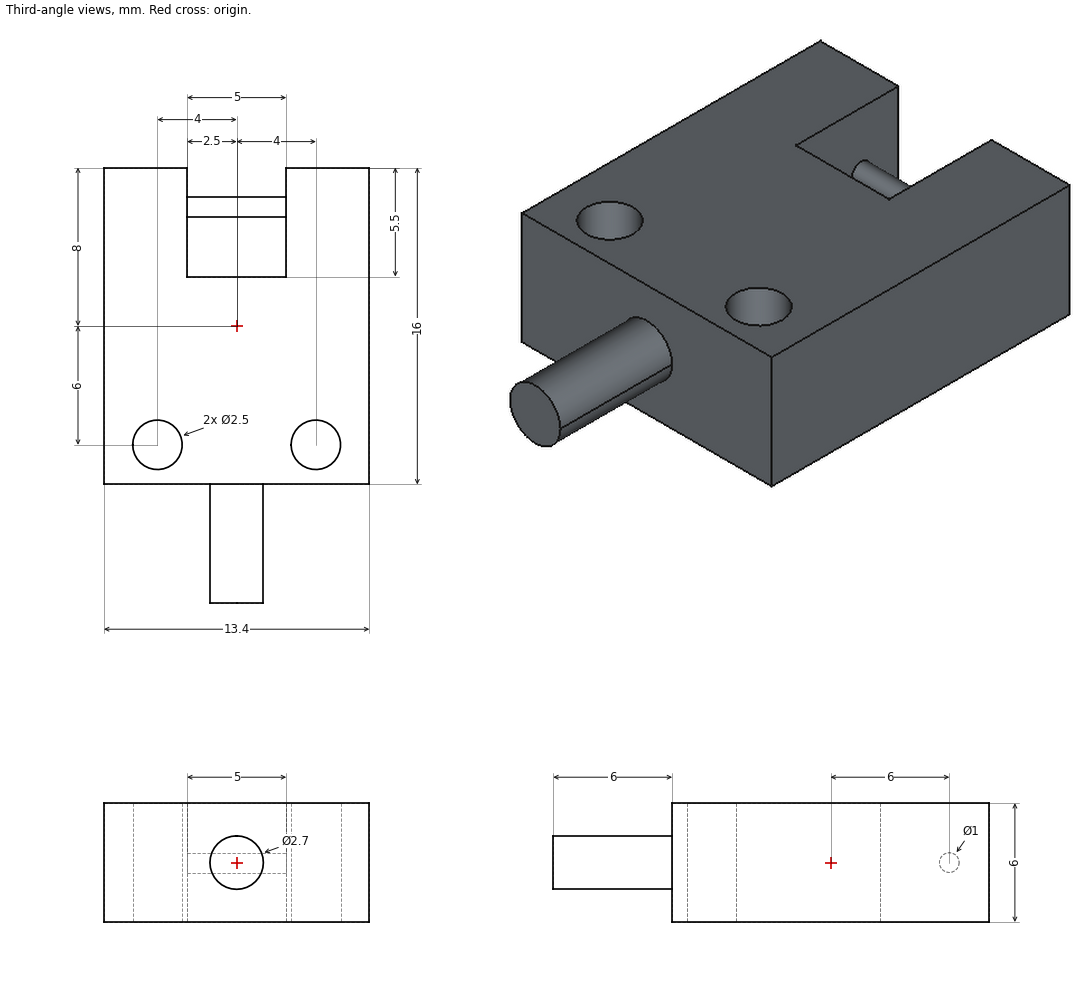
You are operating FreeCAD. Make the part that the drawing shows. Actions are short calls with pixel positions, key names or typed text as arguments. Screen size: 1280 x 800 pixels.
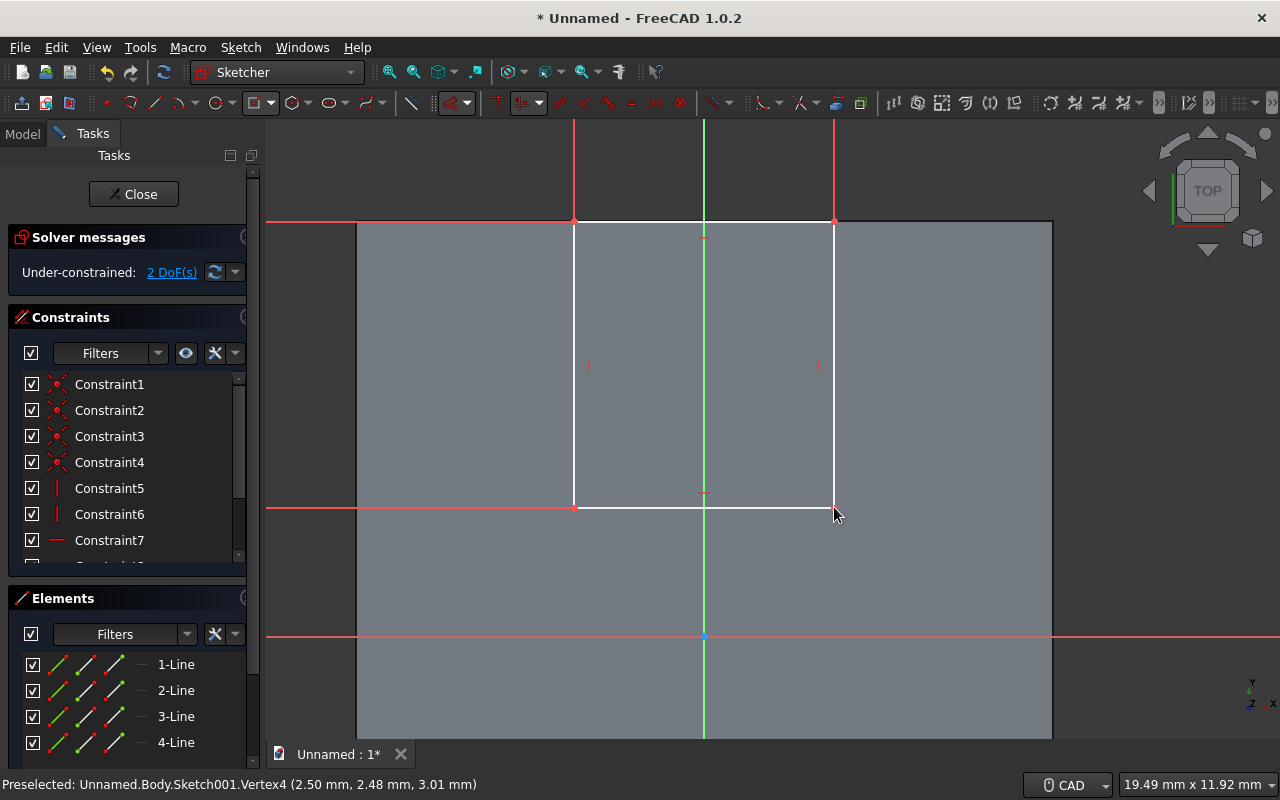
click(450, 104)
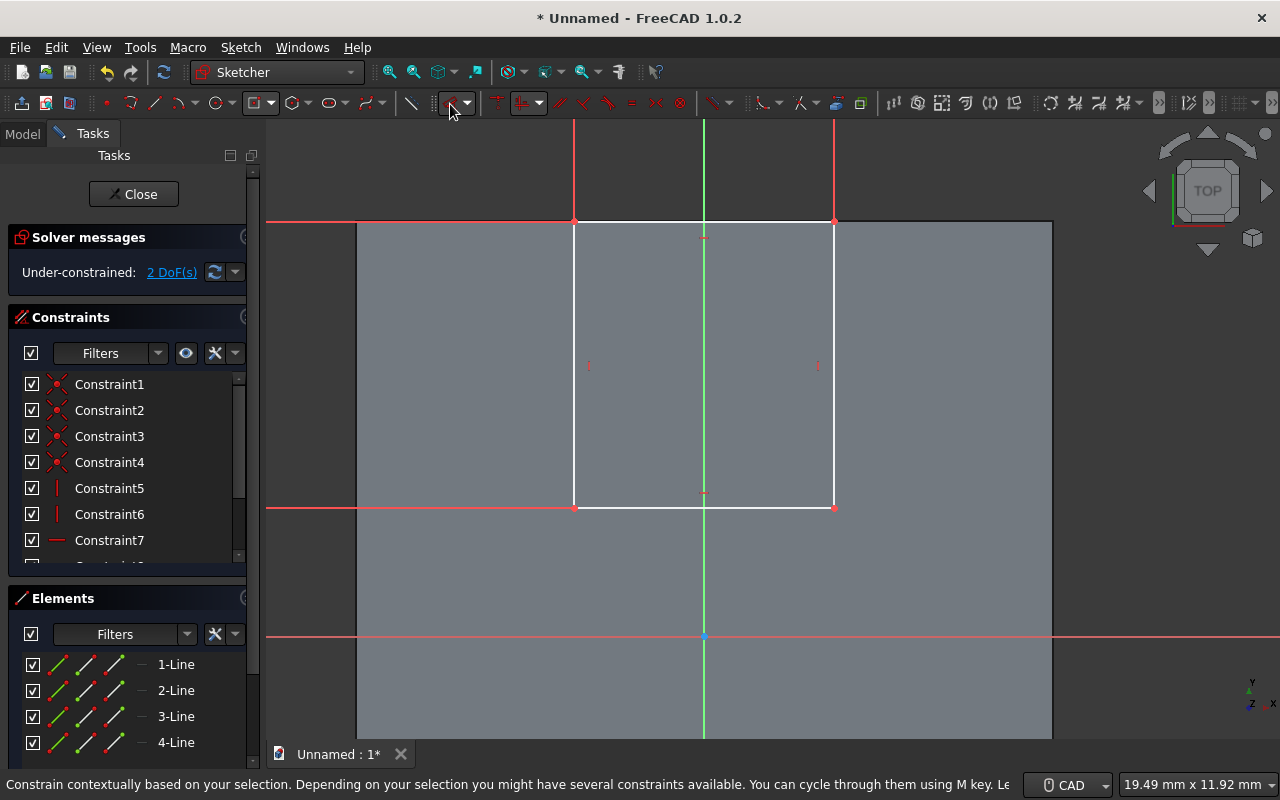
click(574, 222)
click(540, 429)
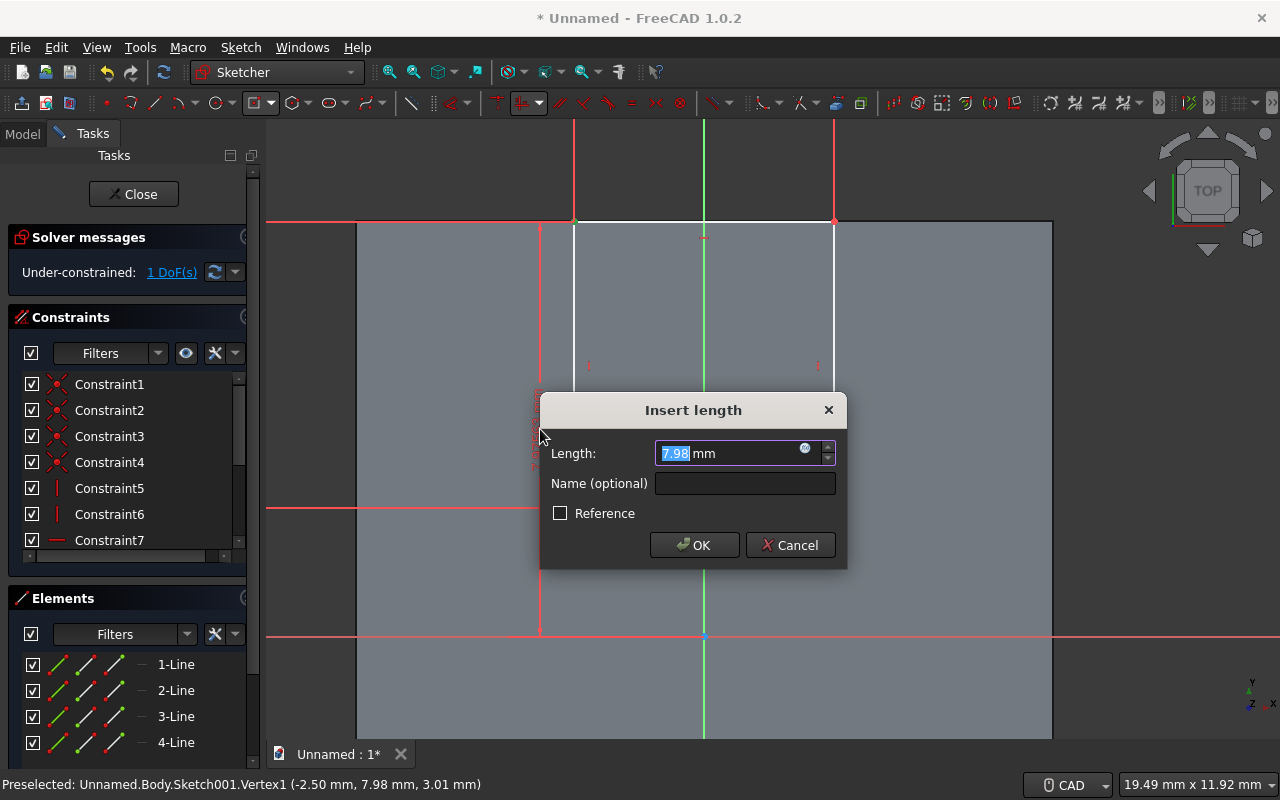
text(8)
key(Return)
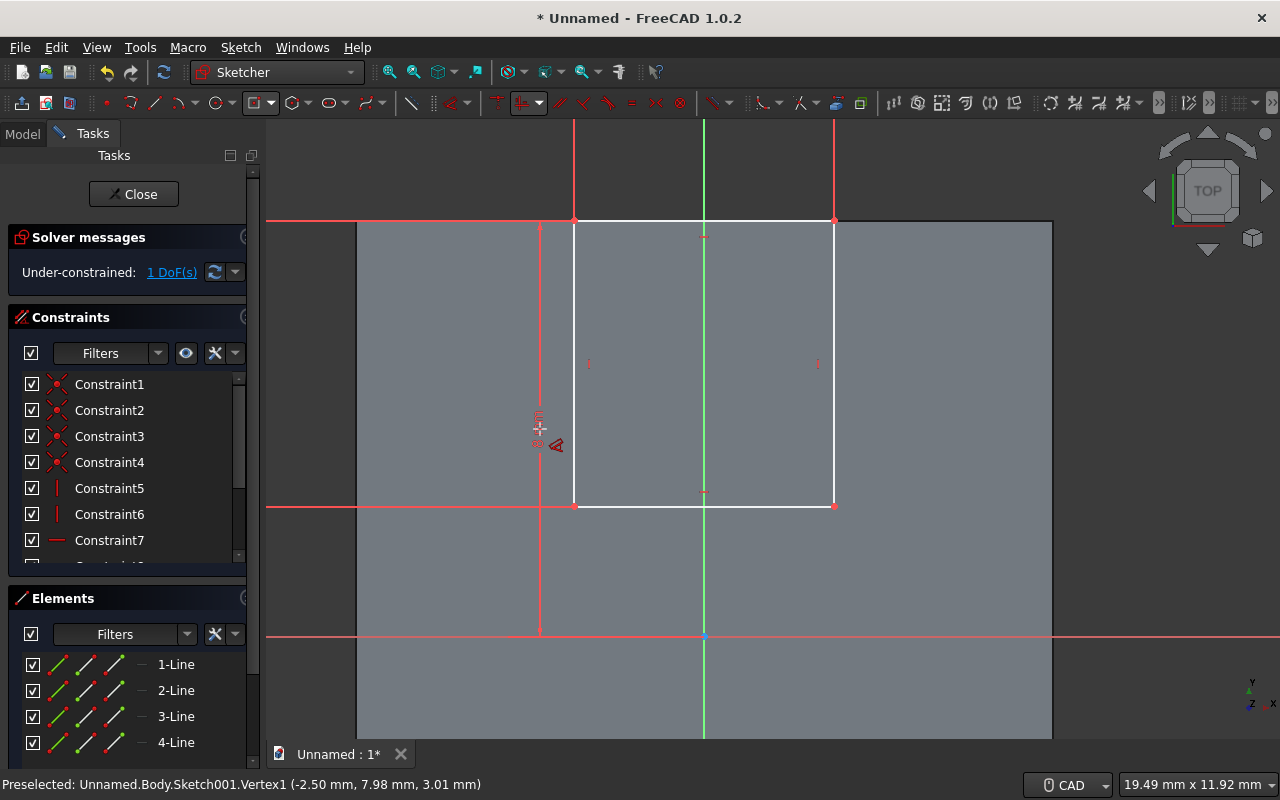
click(574, 221)
click(639, 671)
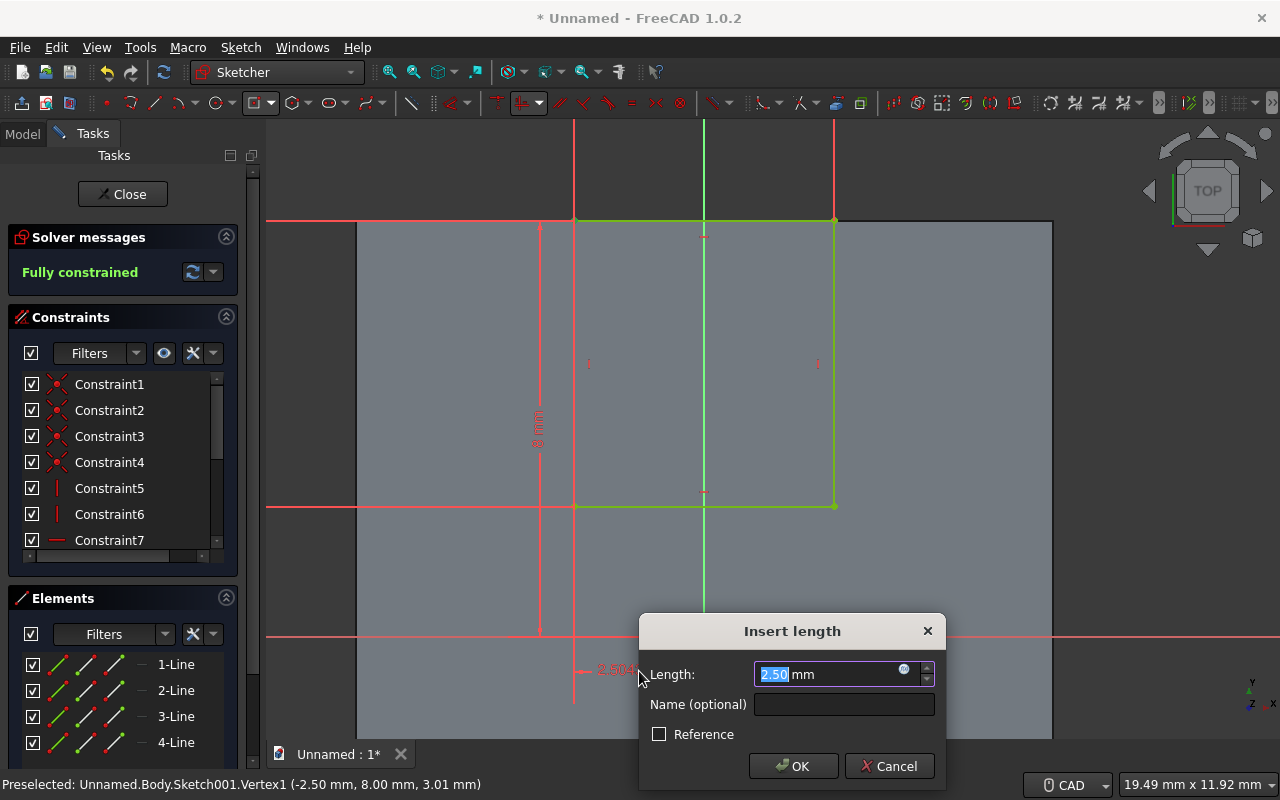
text(2.5)
key(Return)
key(Escape)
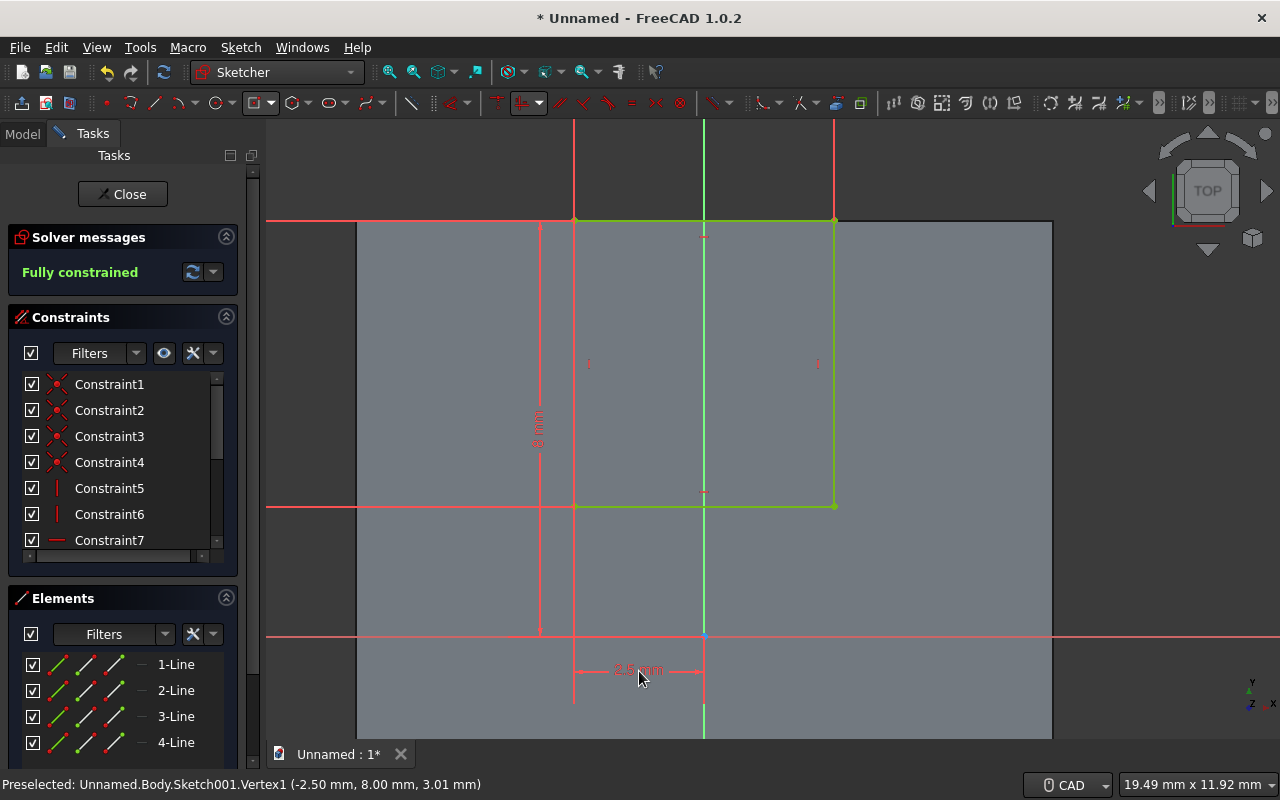
click(123, 194)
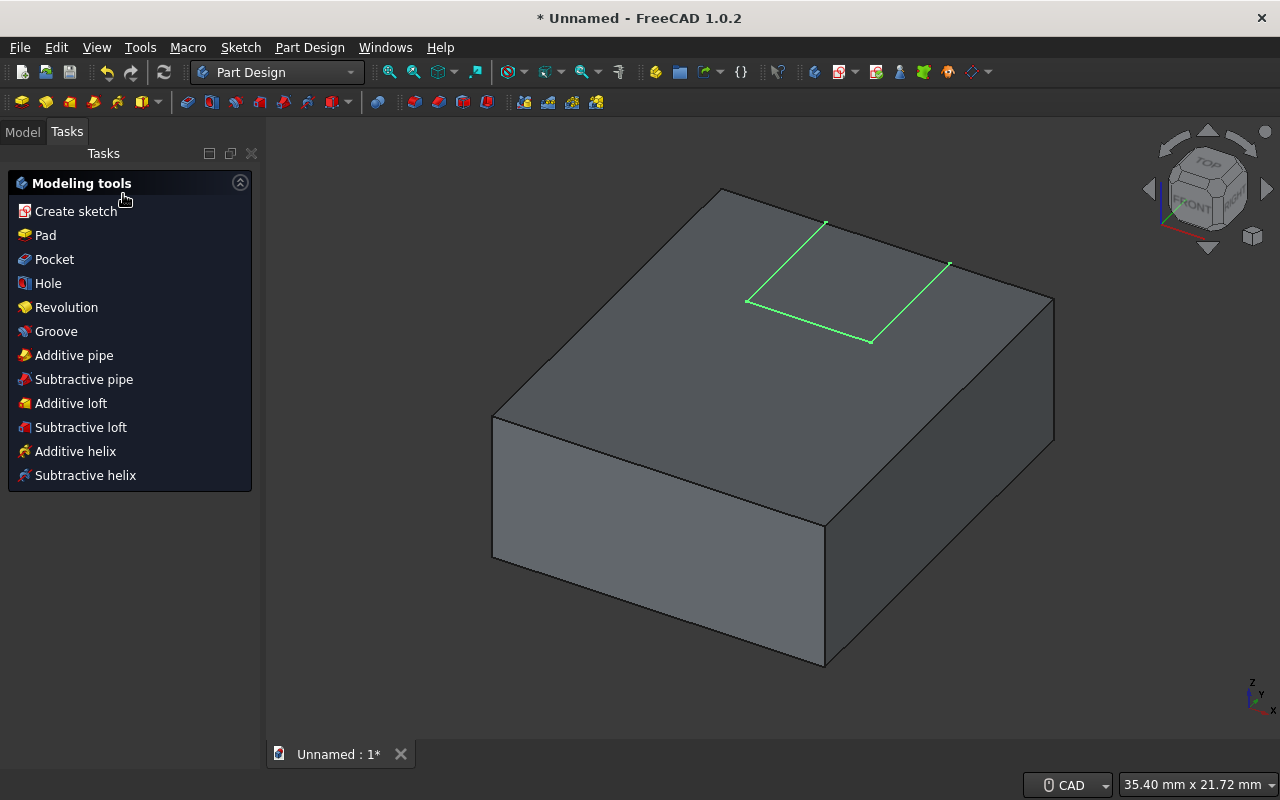
click(188, 102)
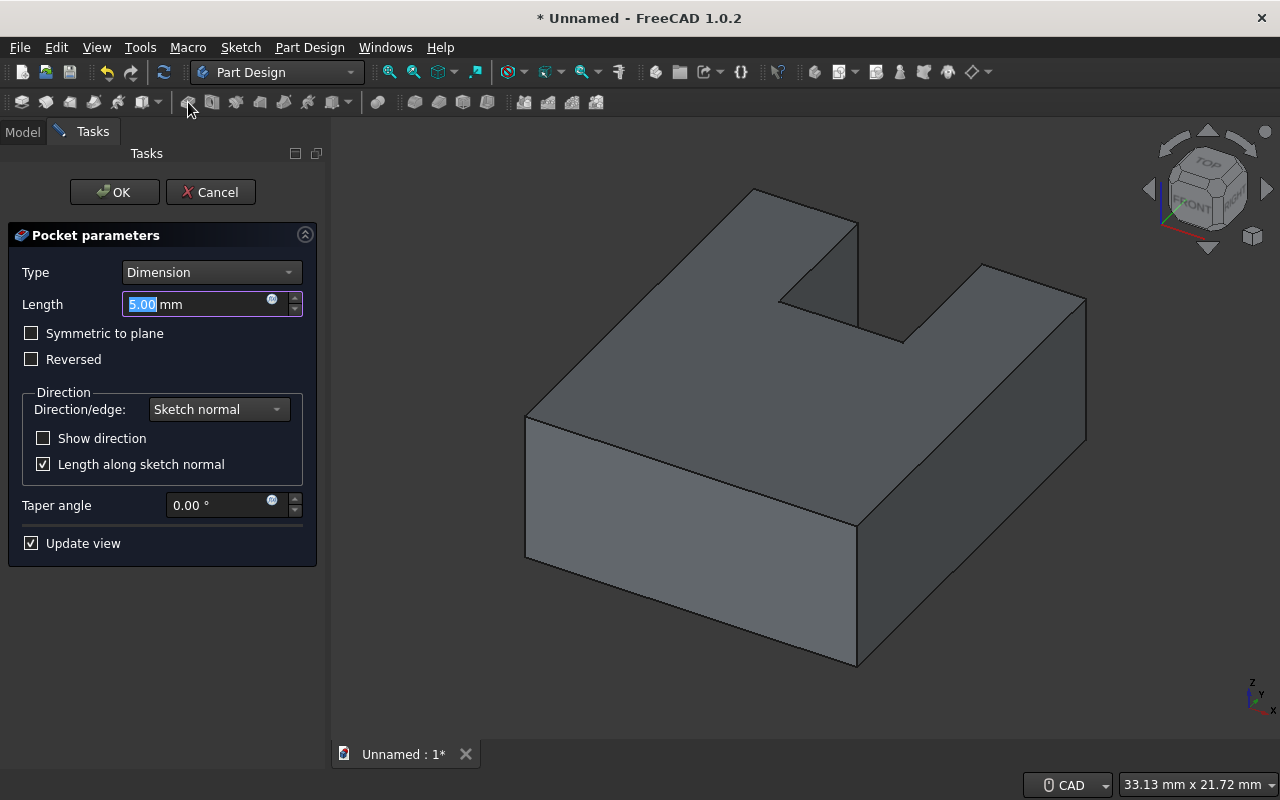
click(212, 272)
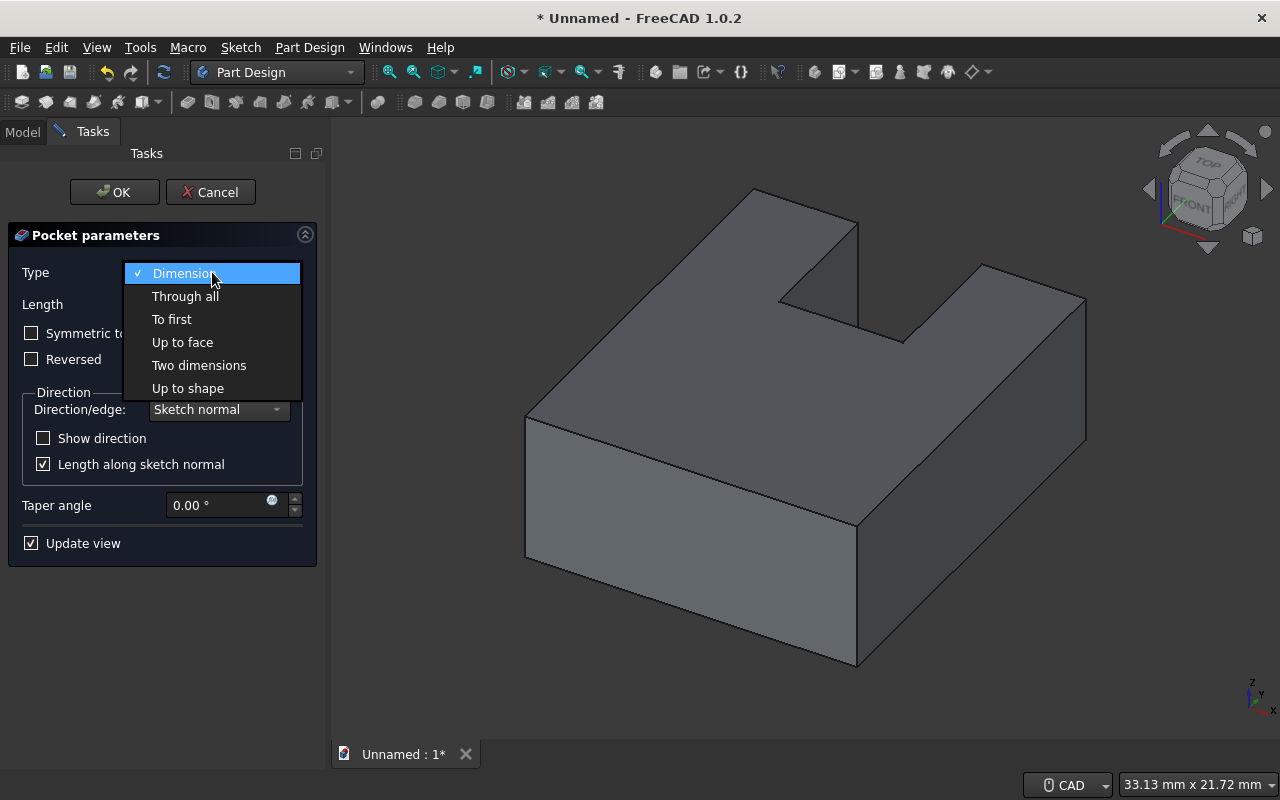
click(212, 296)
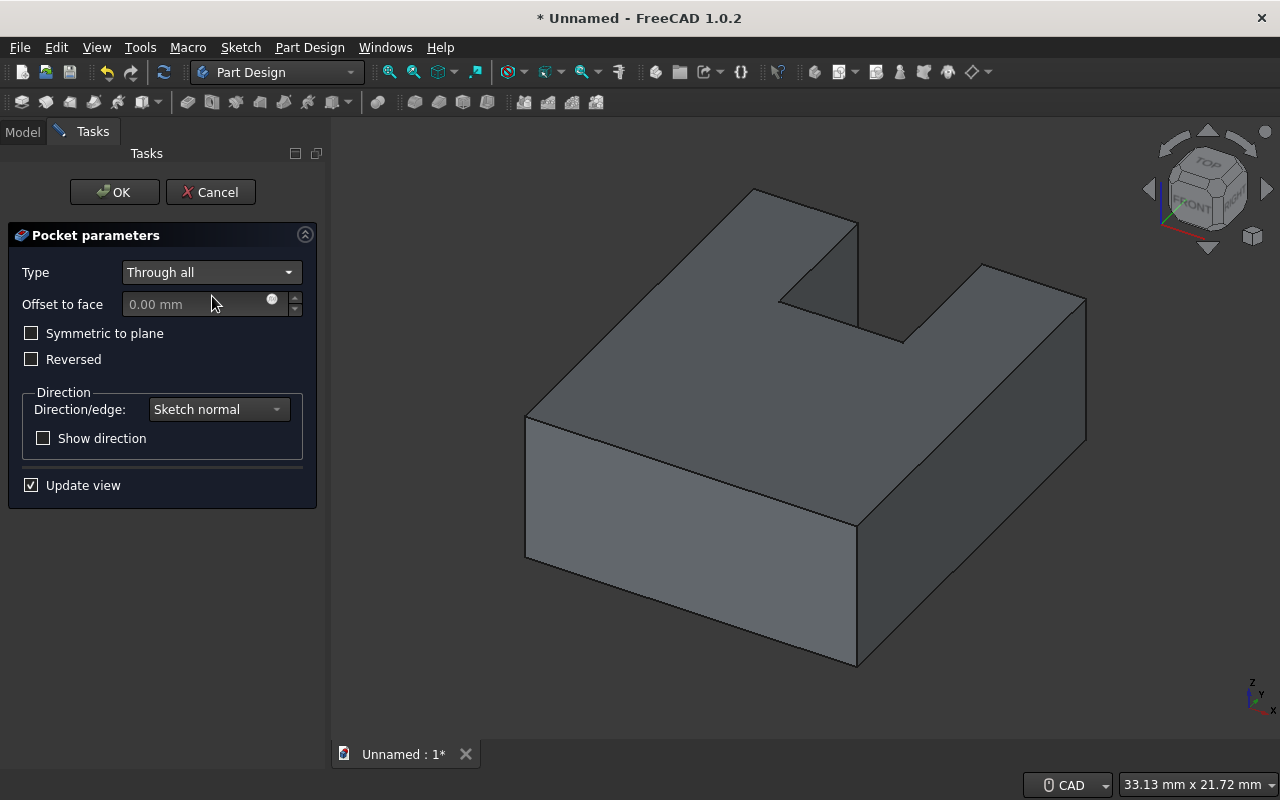
click(115, 192)